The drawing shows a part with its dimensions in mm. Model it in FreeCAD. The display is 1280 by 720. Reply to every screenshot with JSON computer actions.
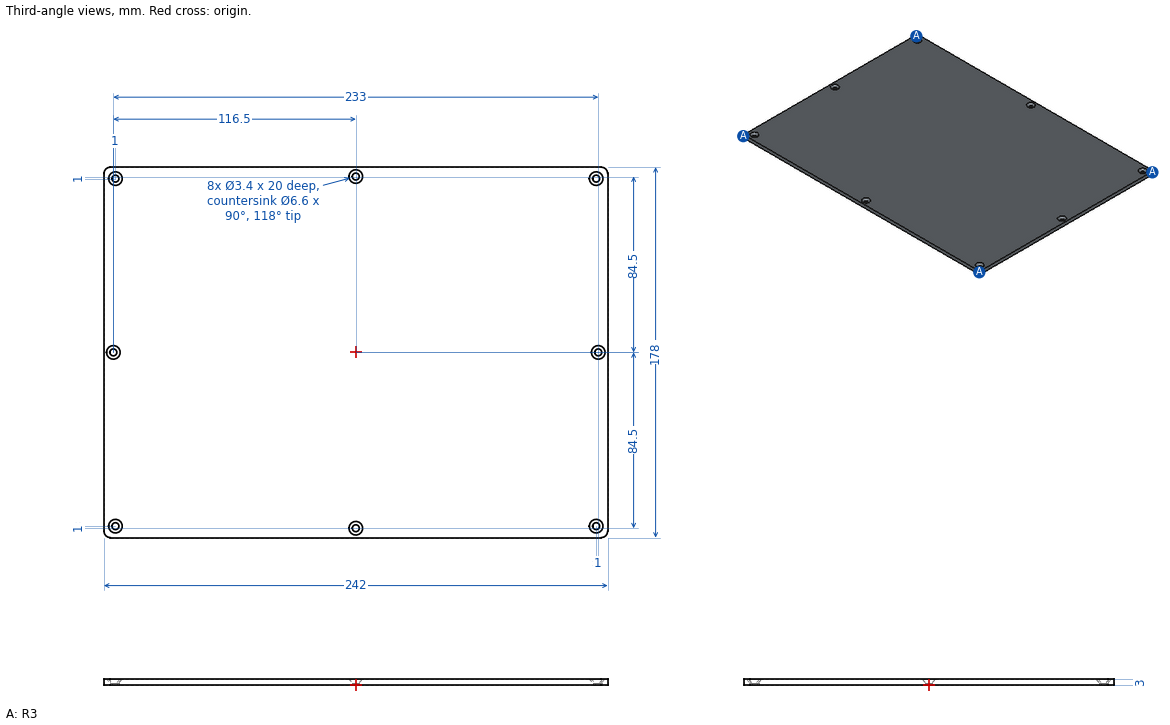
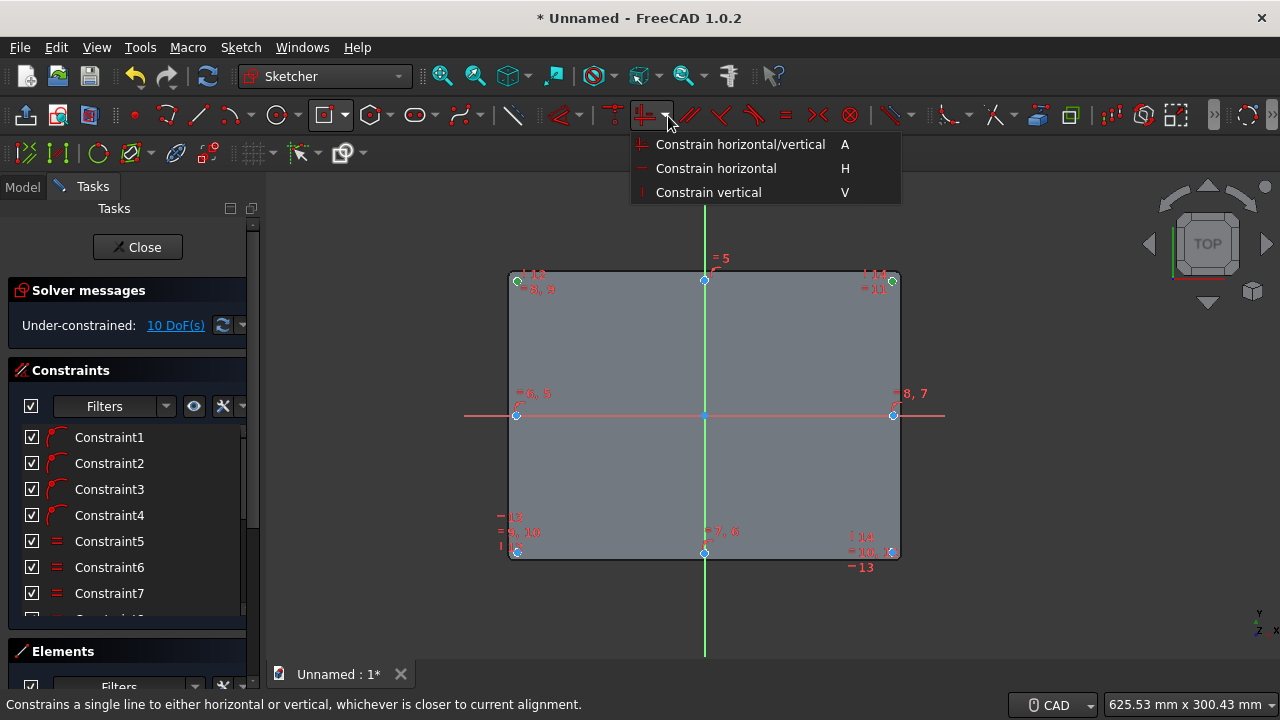
{"action": "left_click", "coordinate": [766, 168]}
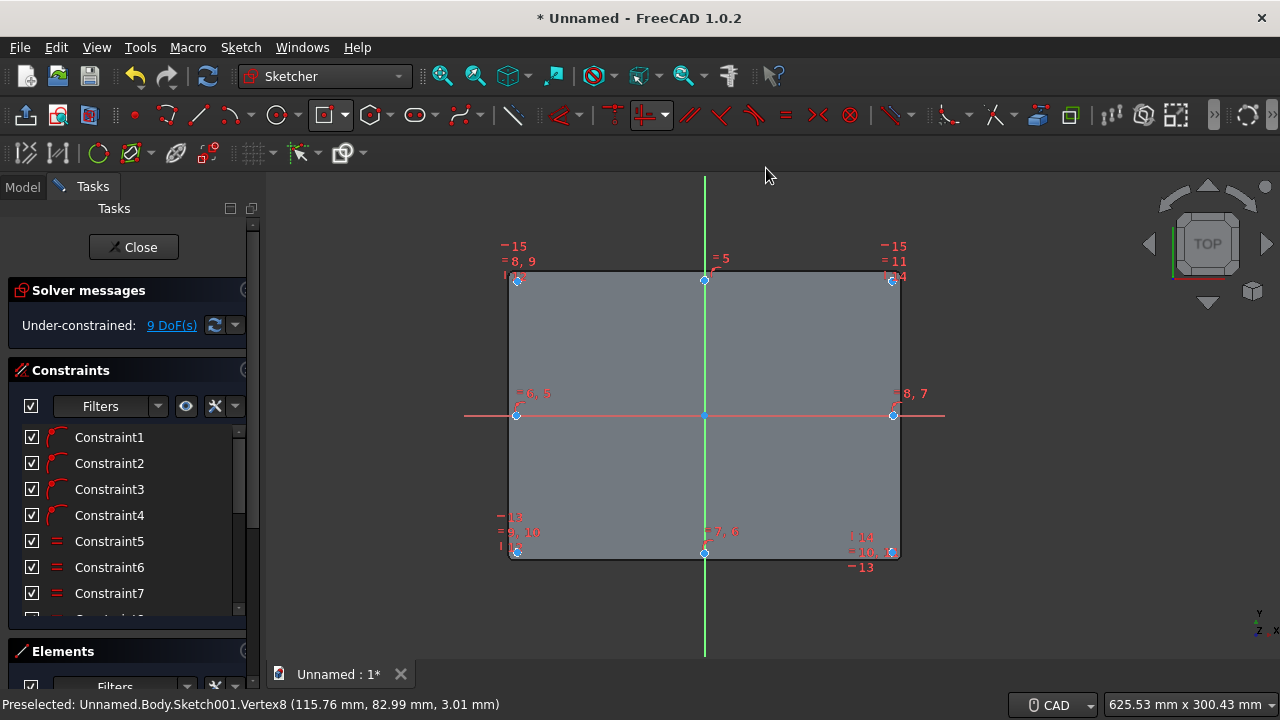
{"action": "scroll", "coordinate": [707, 283], "scroll_direction": "up", "scroll_amount": 10}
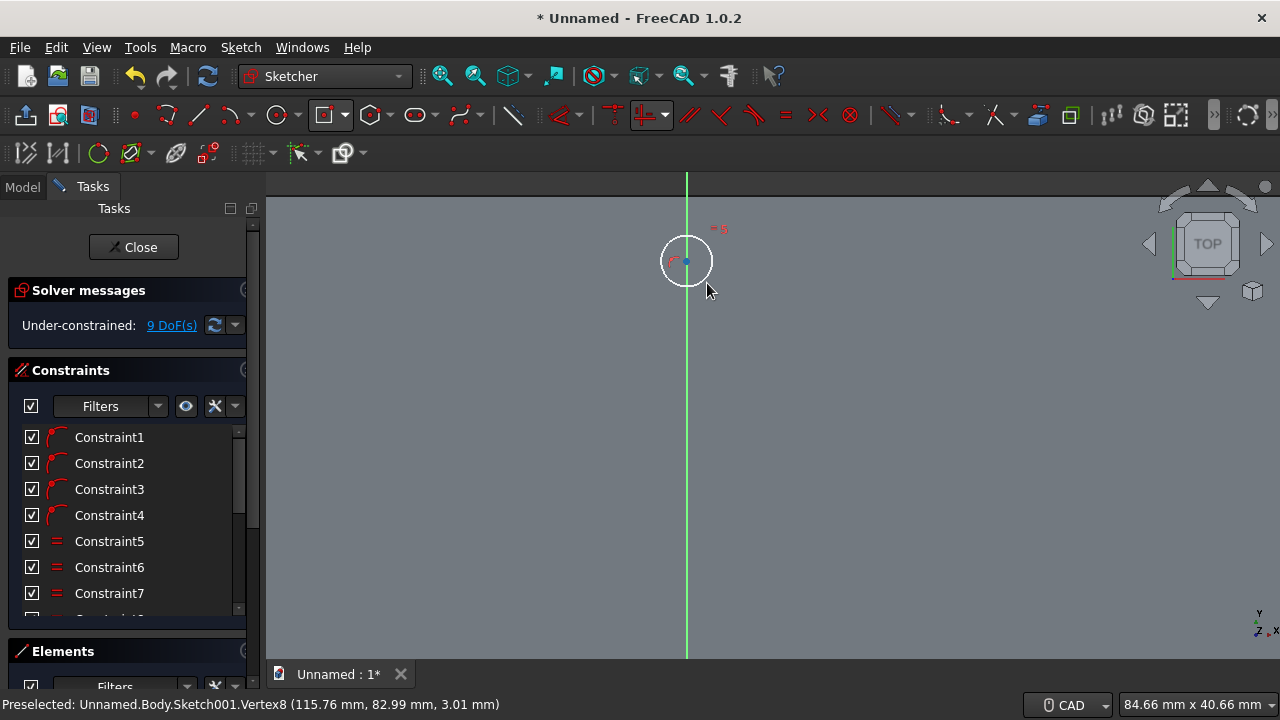
{"action": "left_click", "coordinate": [705, 279]}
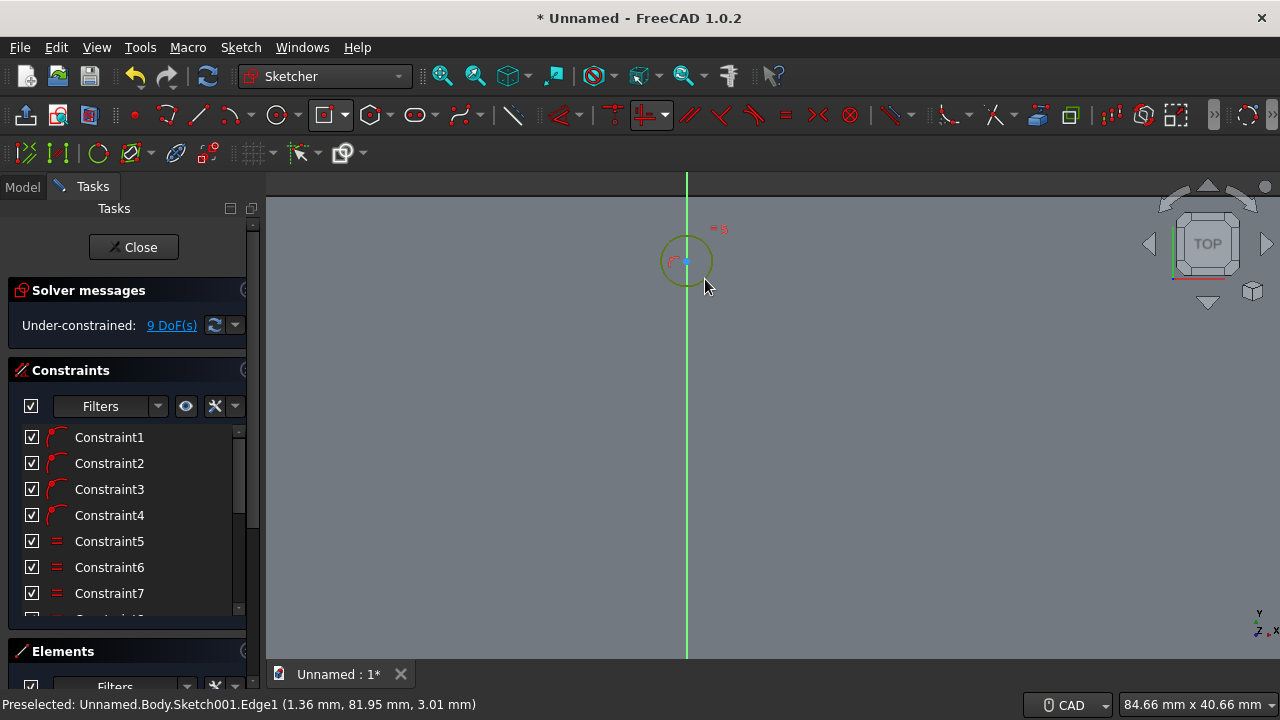
{"action": "key", "text": "k o"}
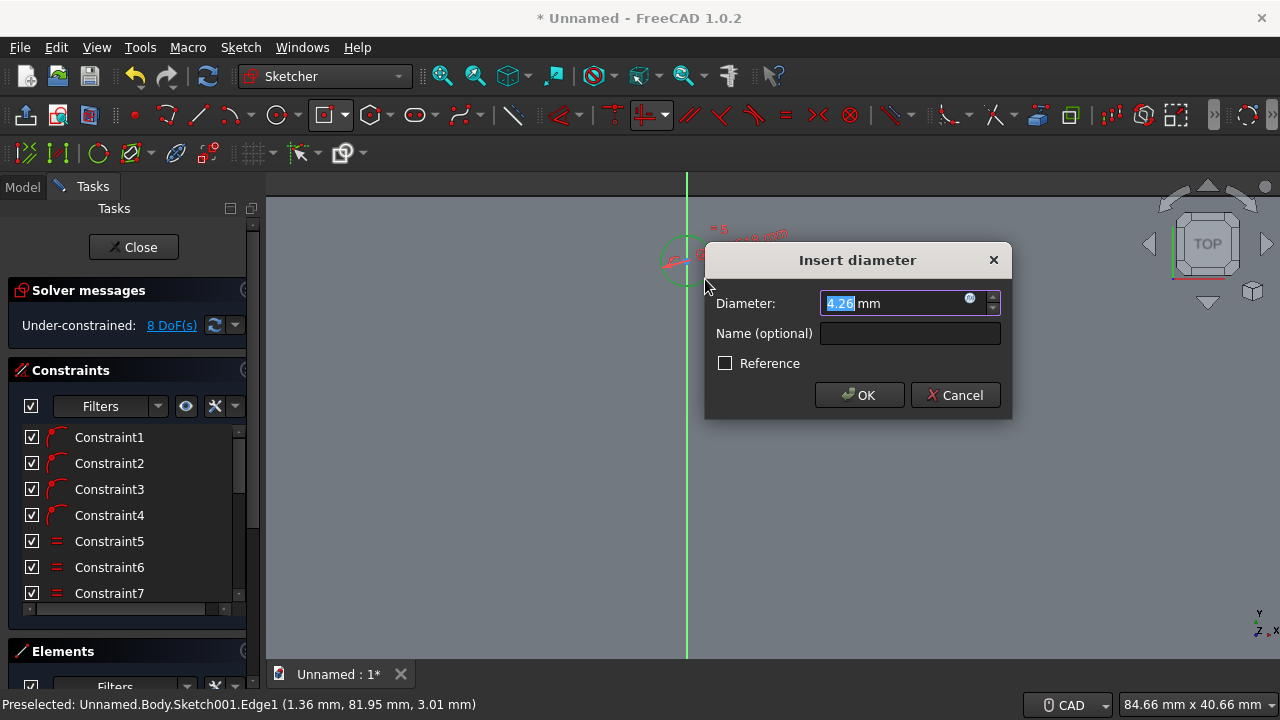
{"action": "type", "text": "3.4"}
{"action": "key", "text": "Return"}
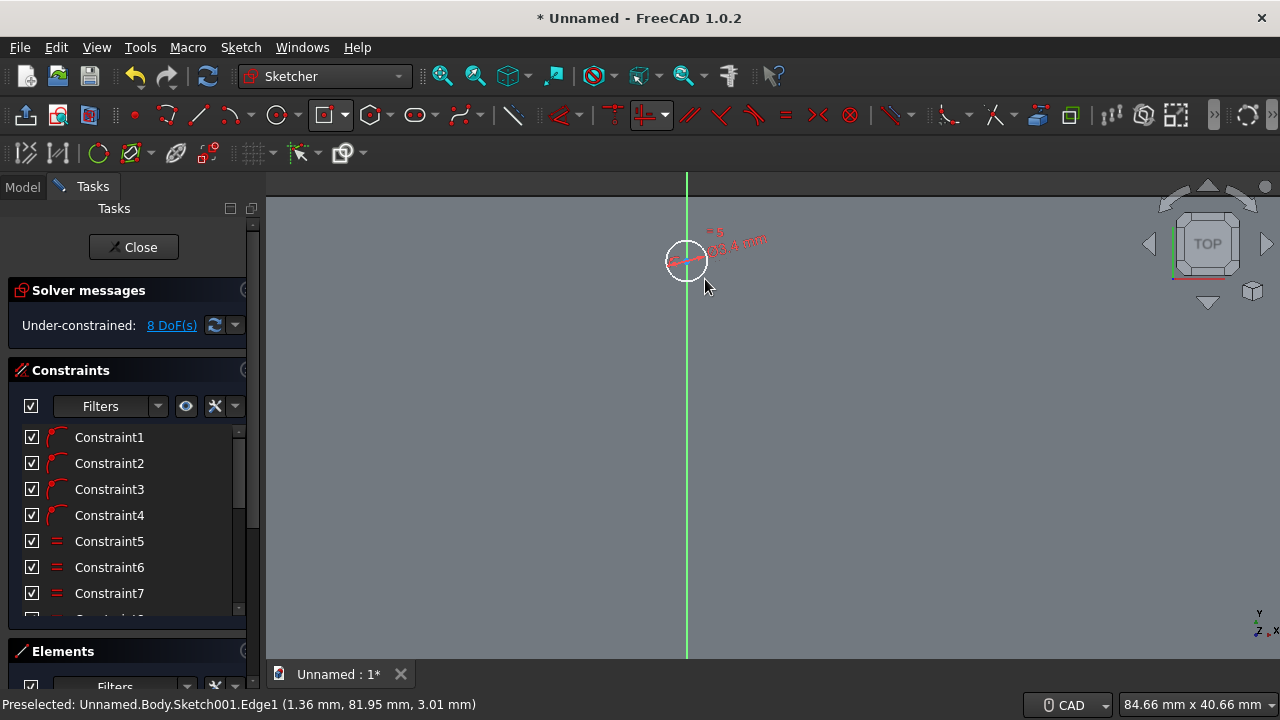
{"action": "scroll", "coordinate": [707, 283], "scroll_direction": "down", "scroll_amount": 10}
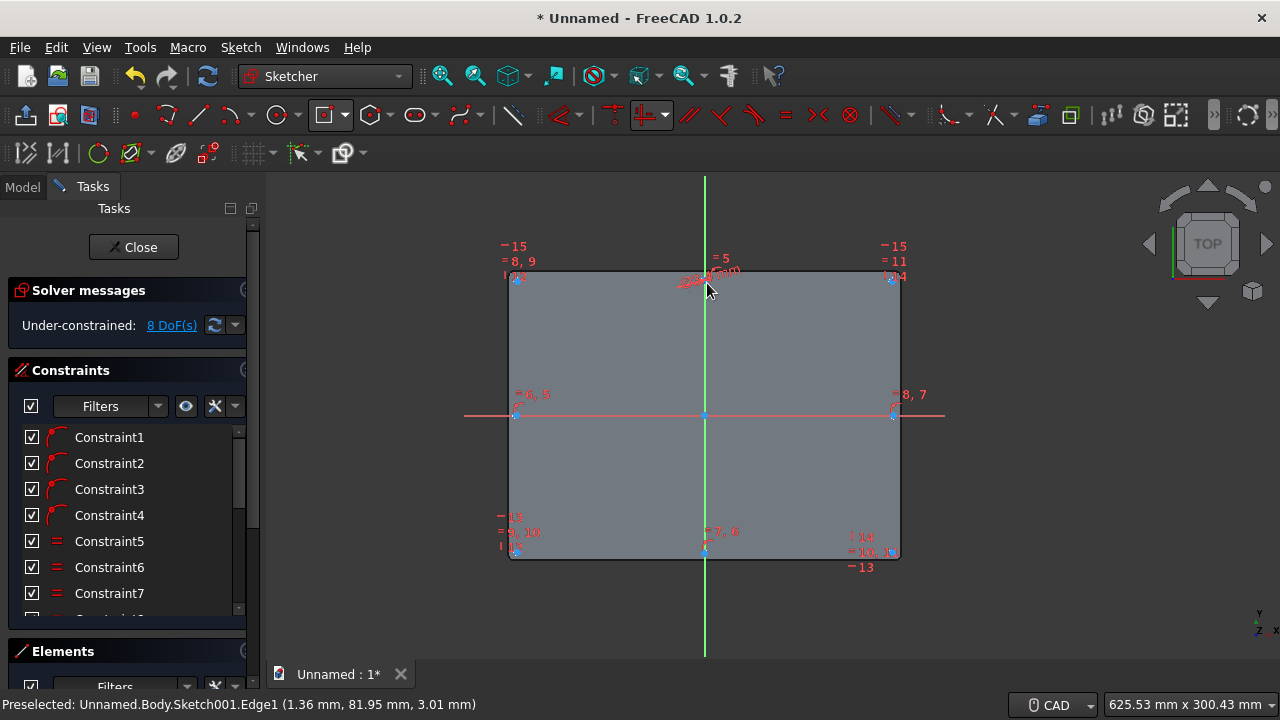
{"action": "scroll", "coordinate": [516, 416], "scroll_direction": "up", "scroll_amount": 16}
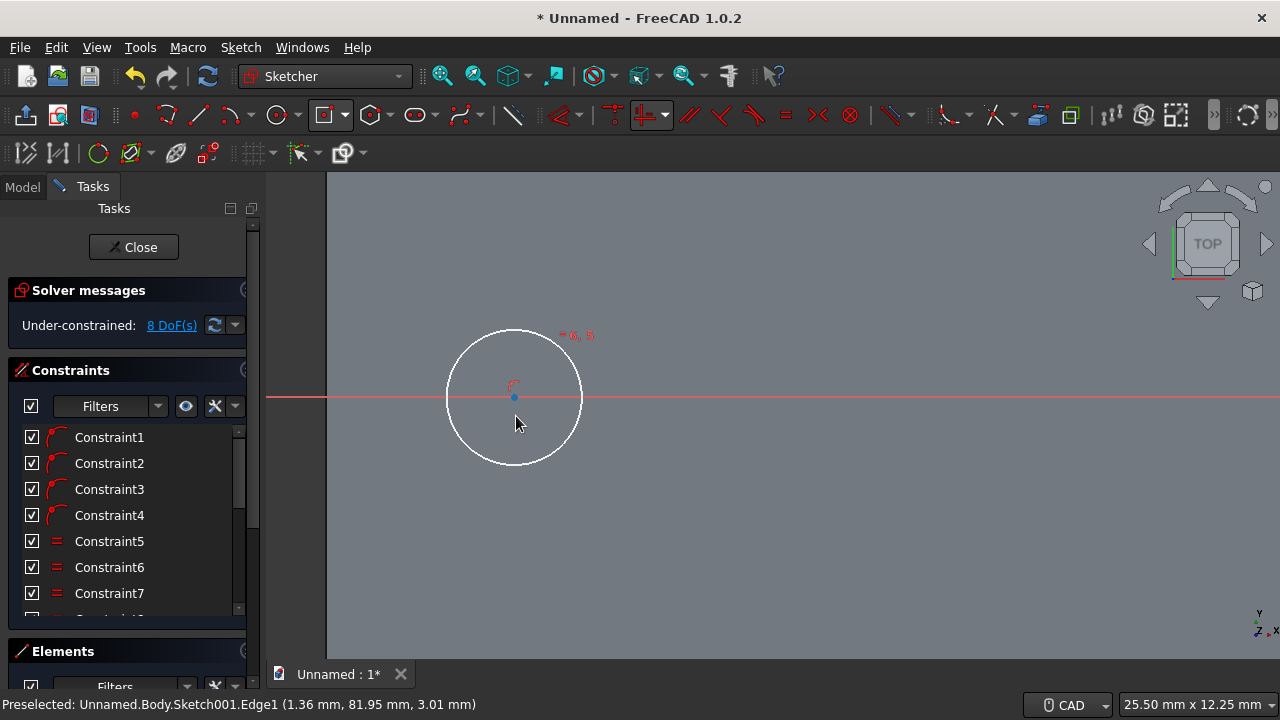
{"action": "left_click", "coordinate": [514, 397]}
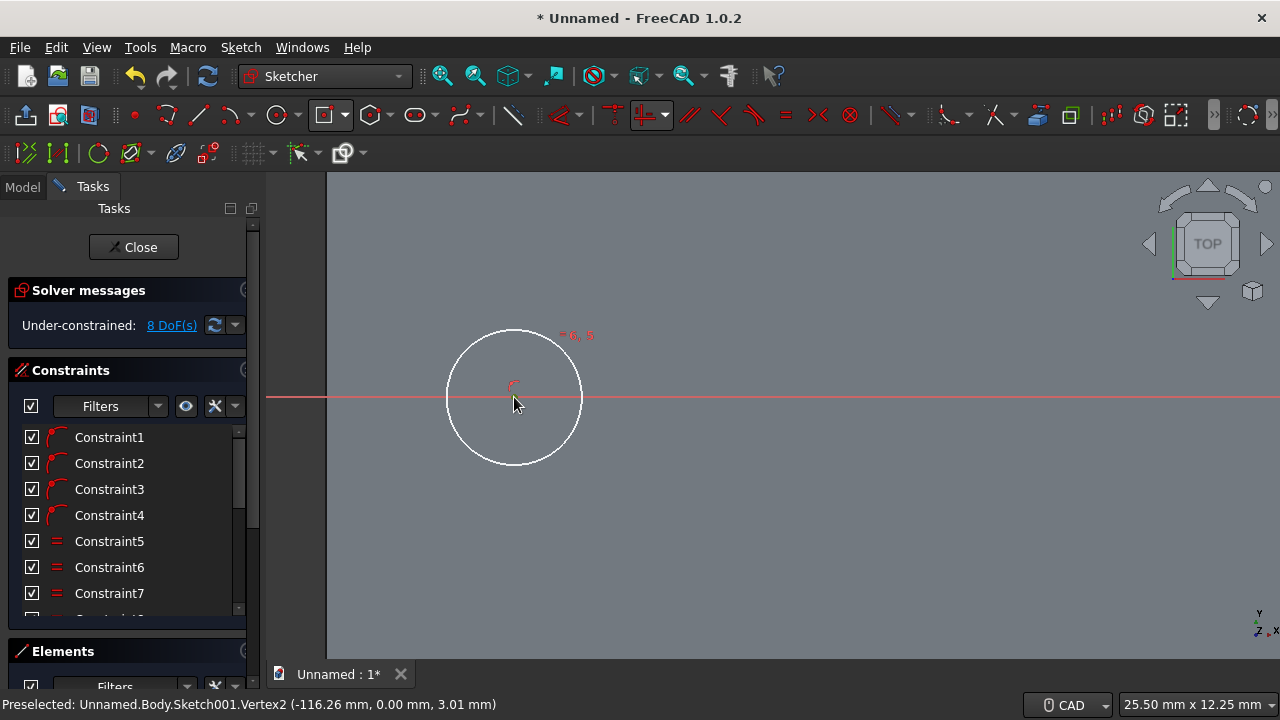
{"action": "scroll", "coordinate": [472, 416], "scroll_direction": "down", "scroll_amount": 15}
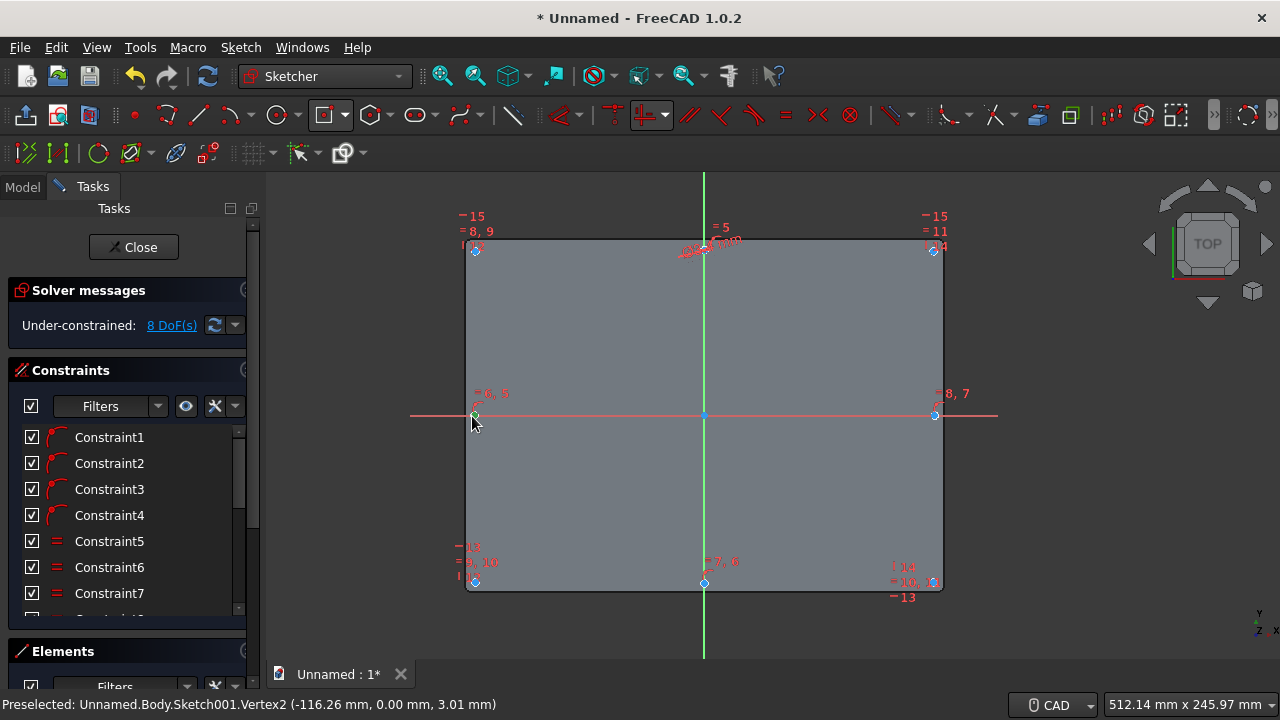
{"action": "scroll", "coordinate": [476, 251], "scroll_direction": "up", "scroll_amount": 15}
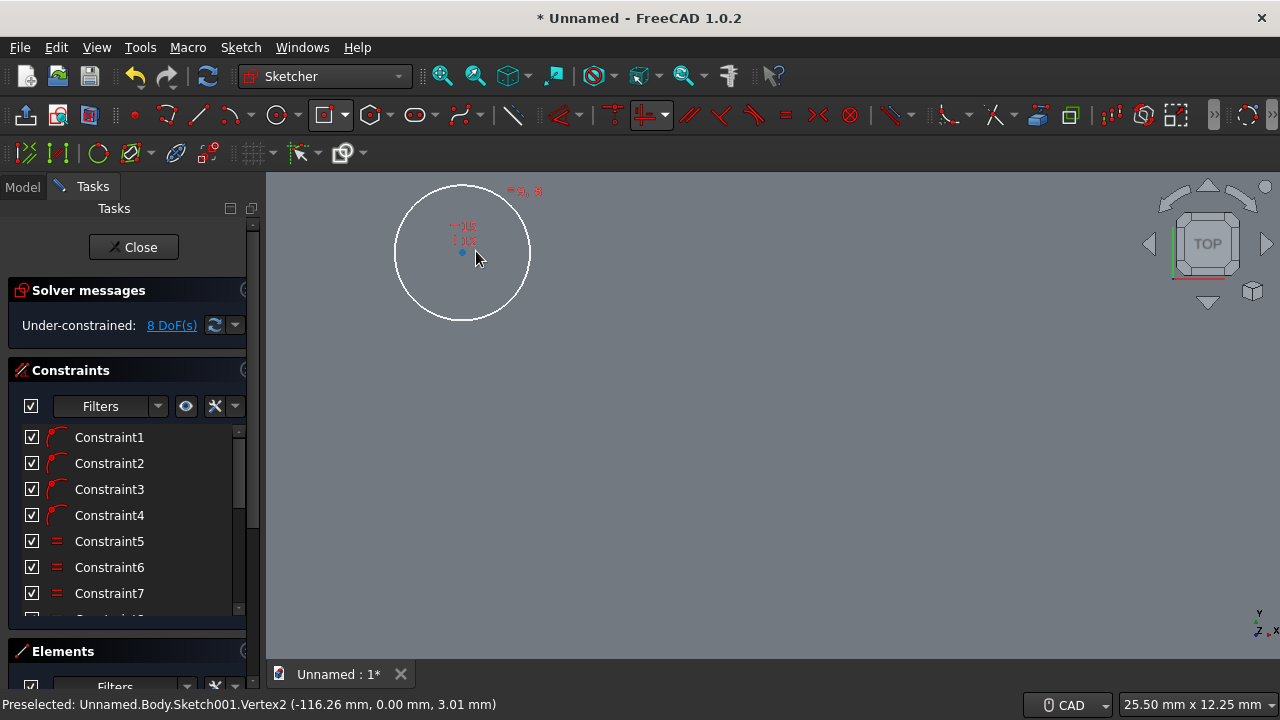
{"action": "left_click", "coordinate": [462, 253]}